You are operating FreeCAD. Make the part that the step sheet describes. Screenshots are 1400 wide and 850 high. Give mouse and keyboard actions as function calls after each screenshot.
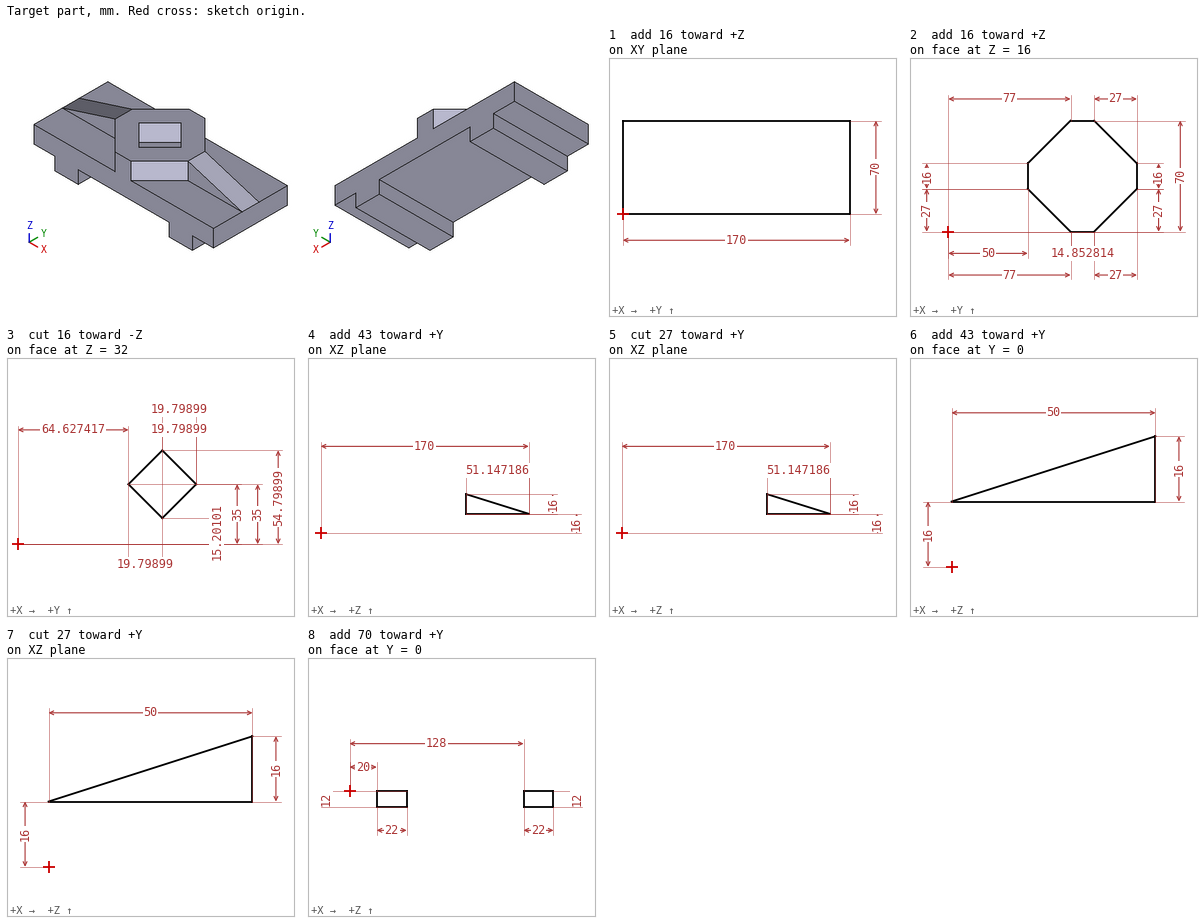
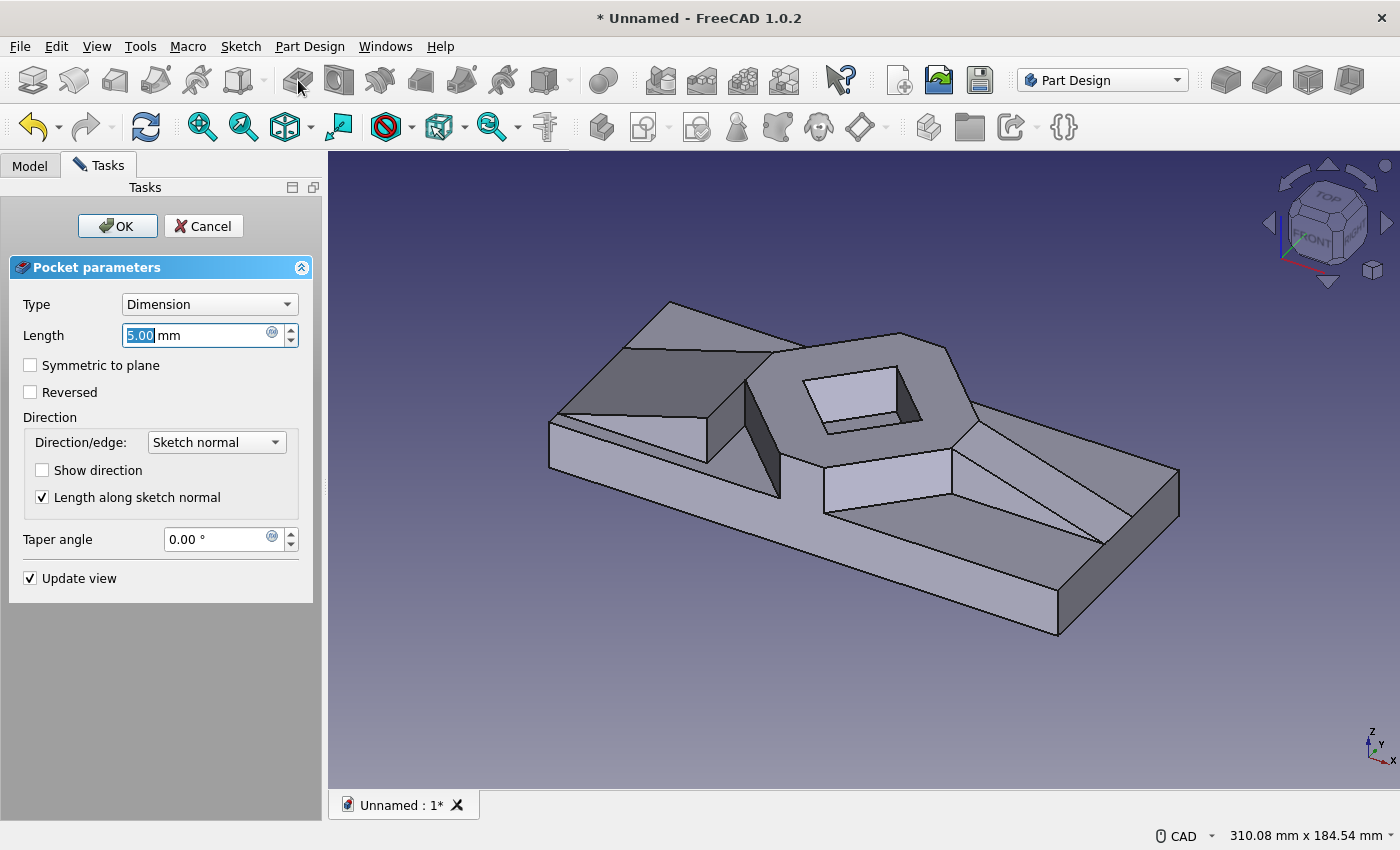
text(27)
key(Tab)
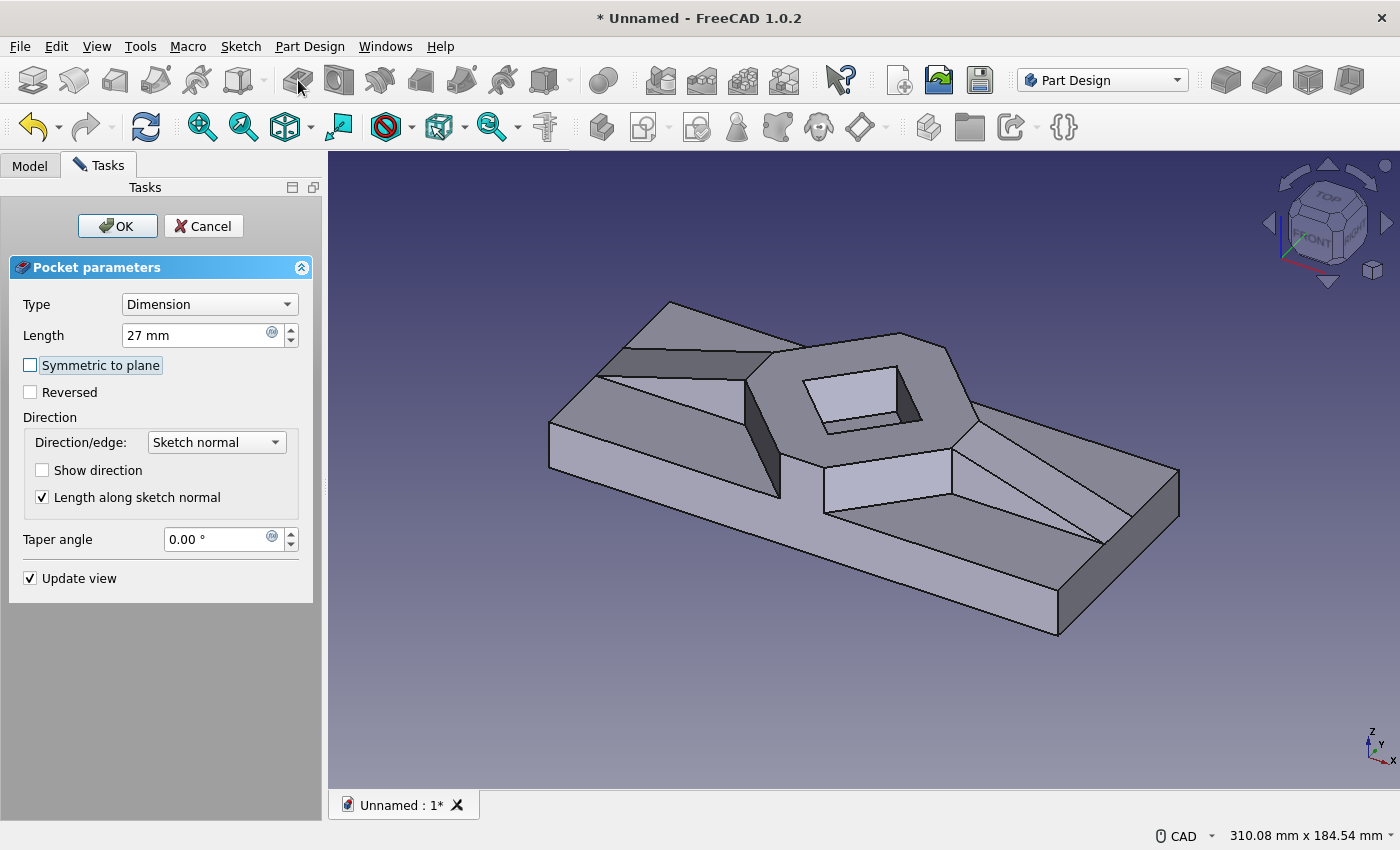
click(118, 226)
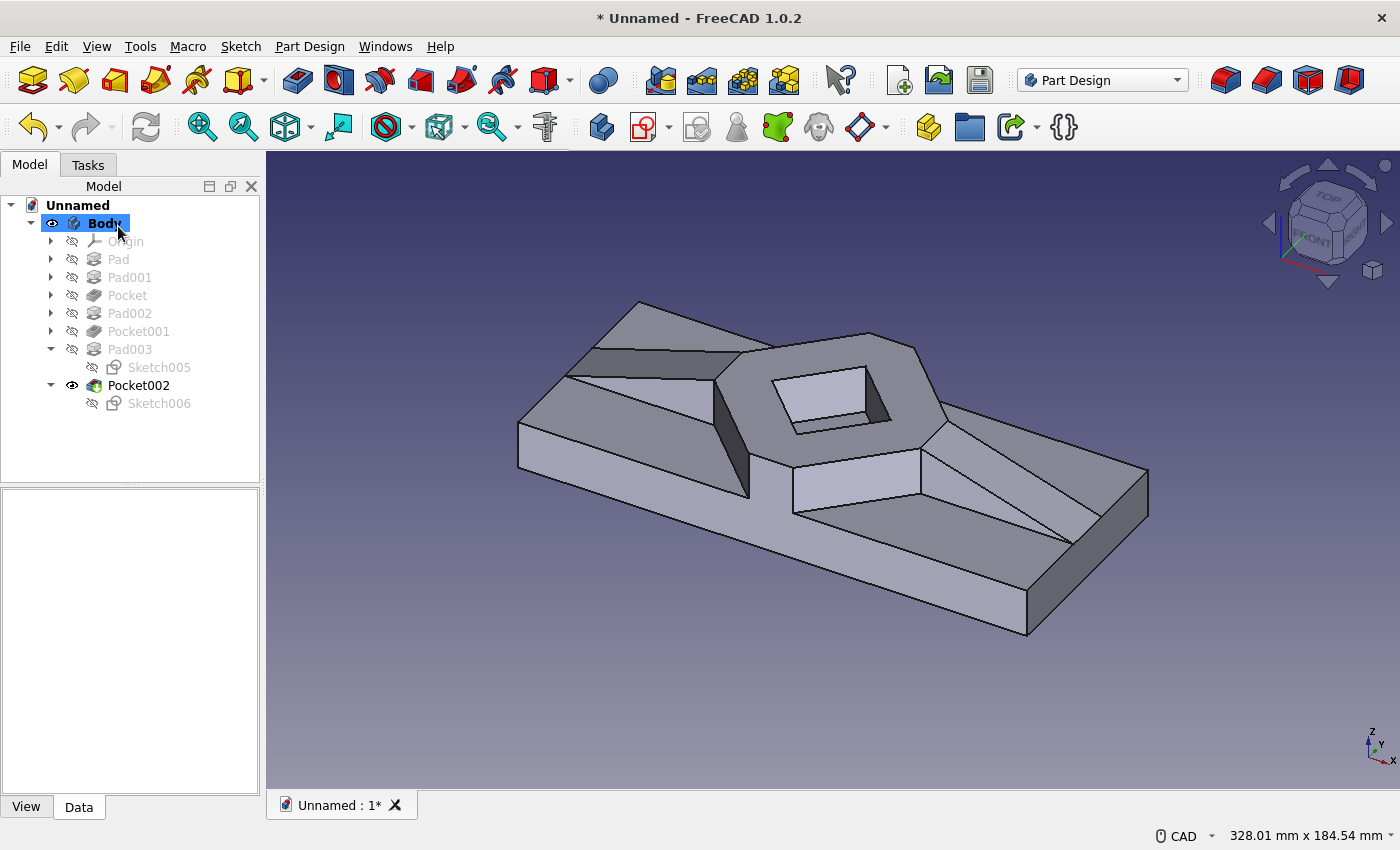
click(772, 518)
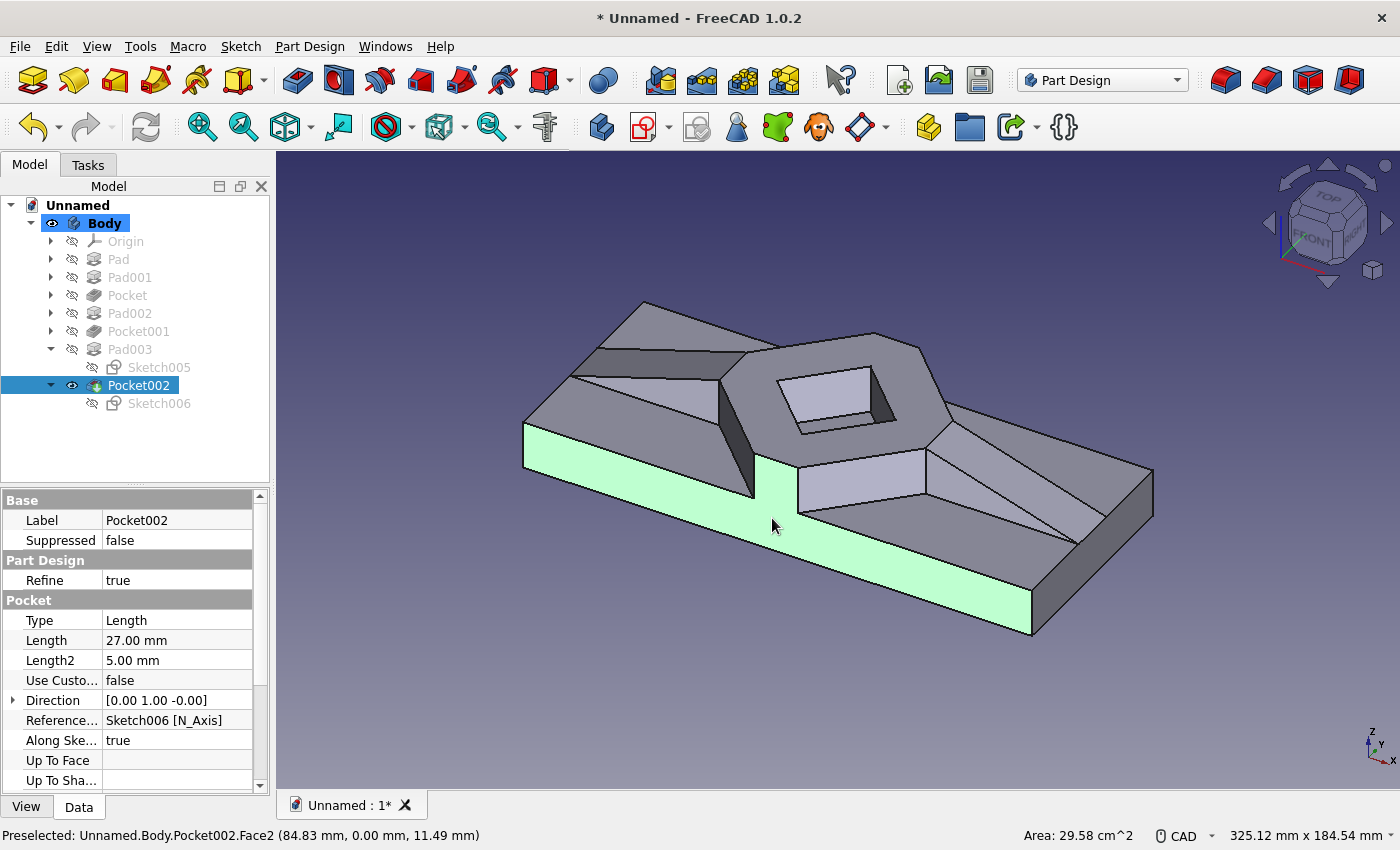
click(642, 128)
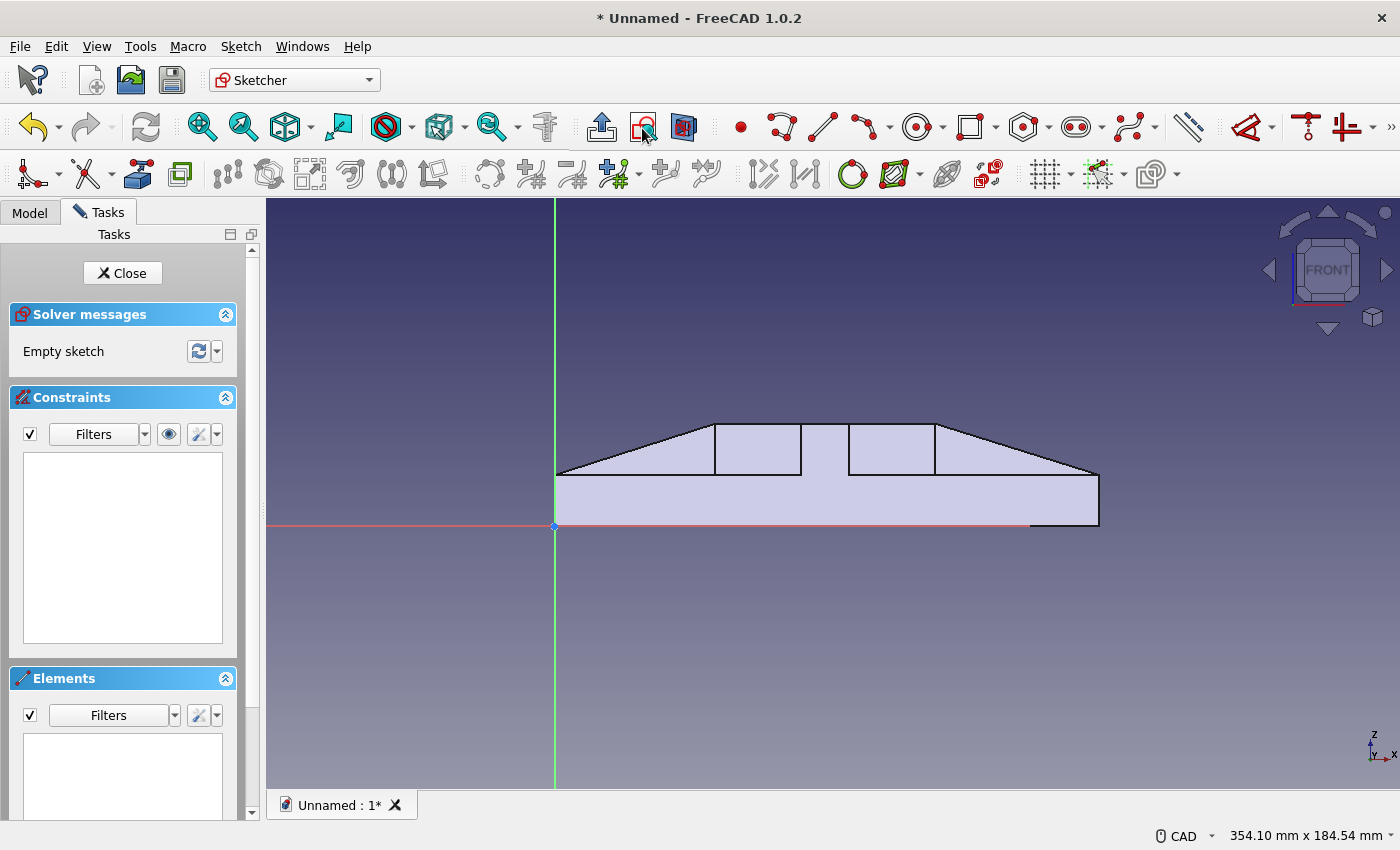
scroll(857, 651, up, 2)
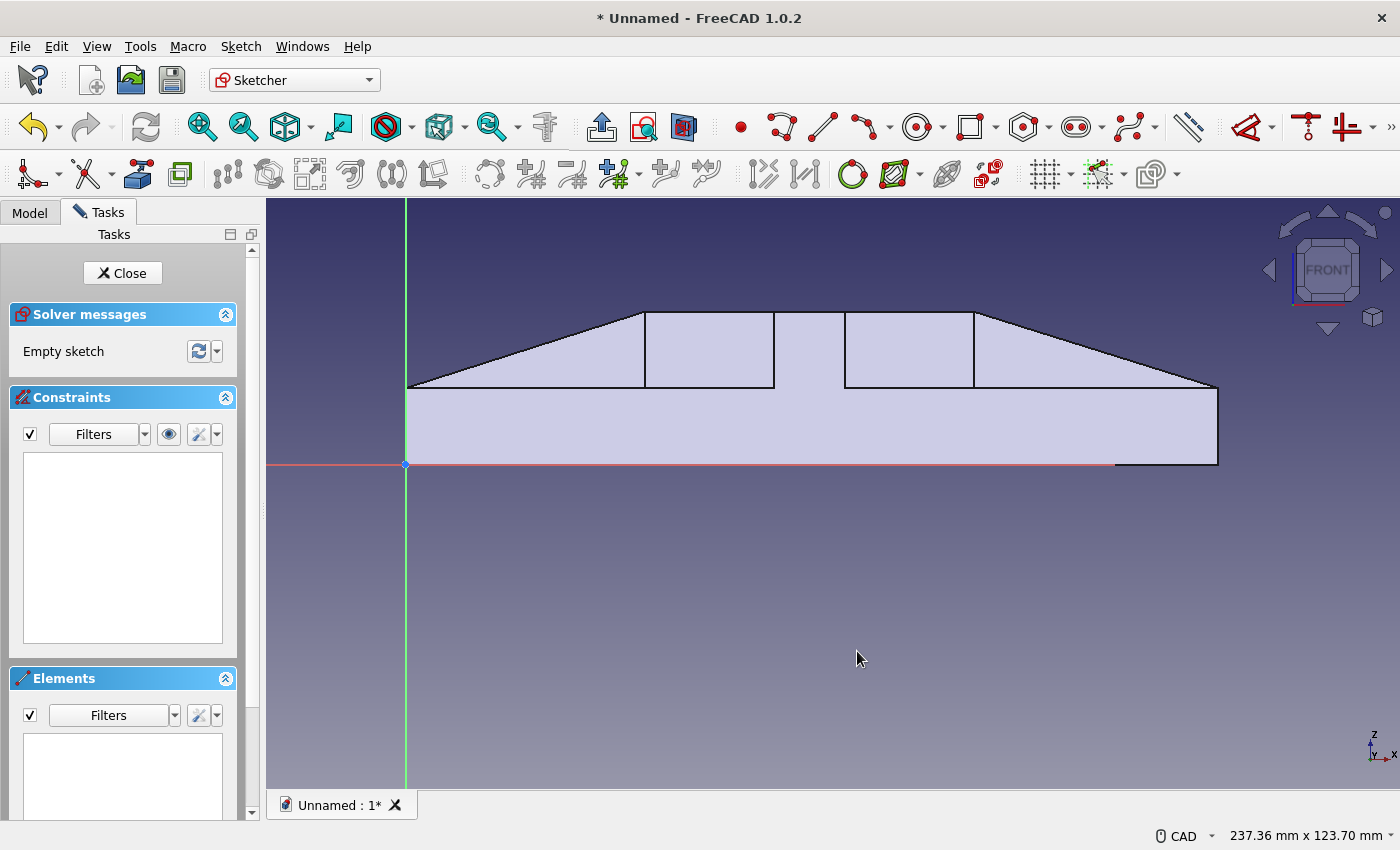
key(g)
key(r)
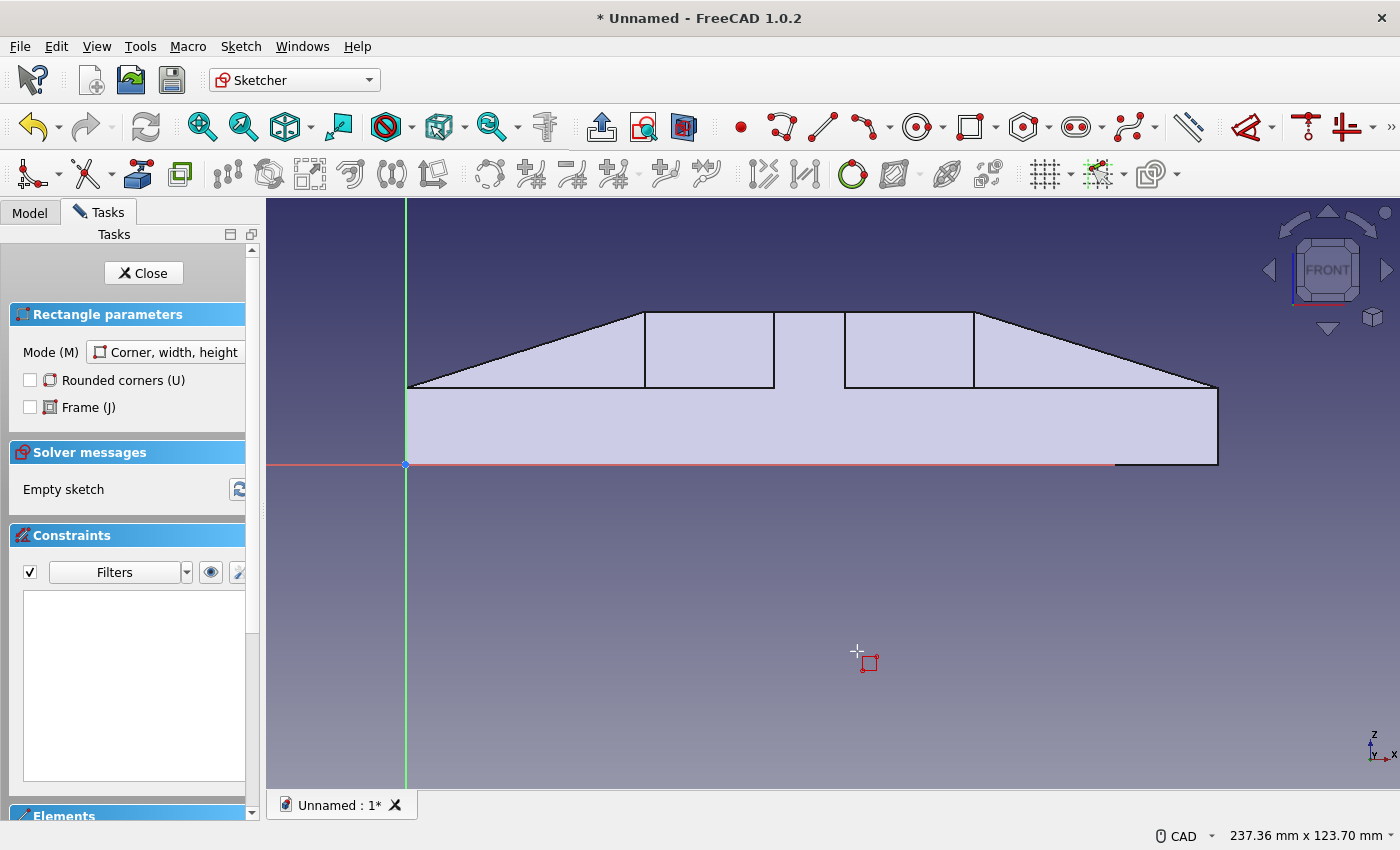
click(501, 465)
move(607, 522)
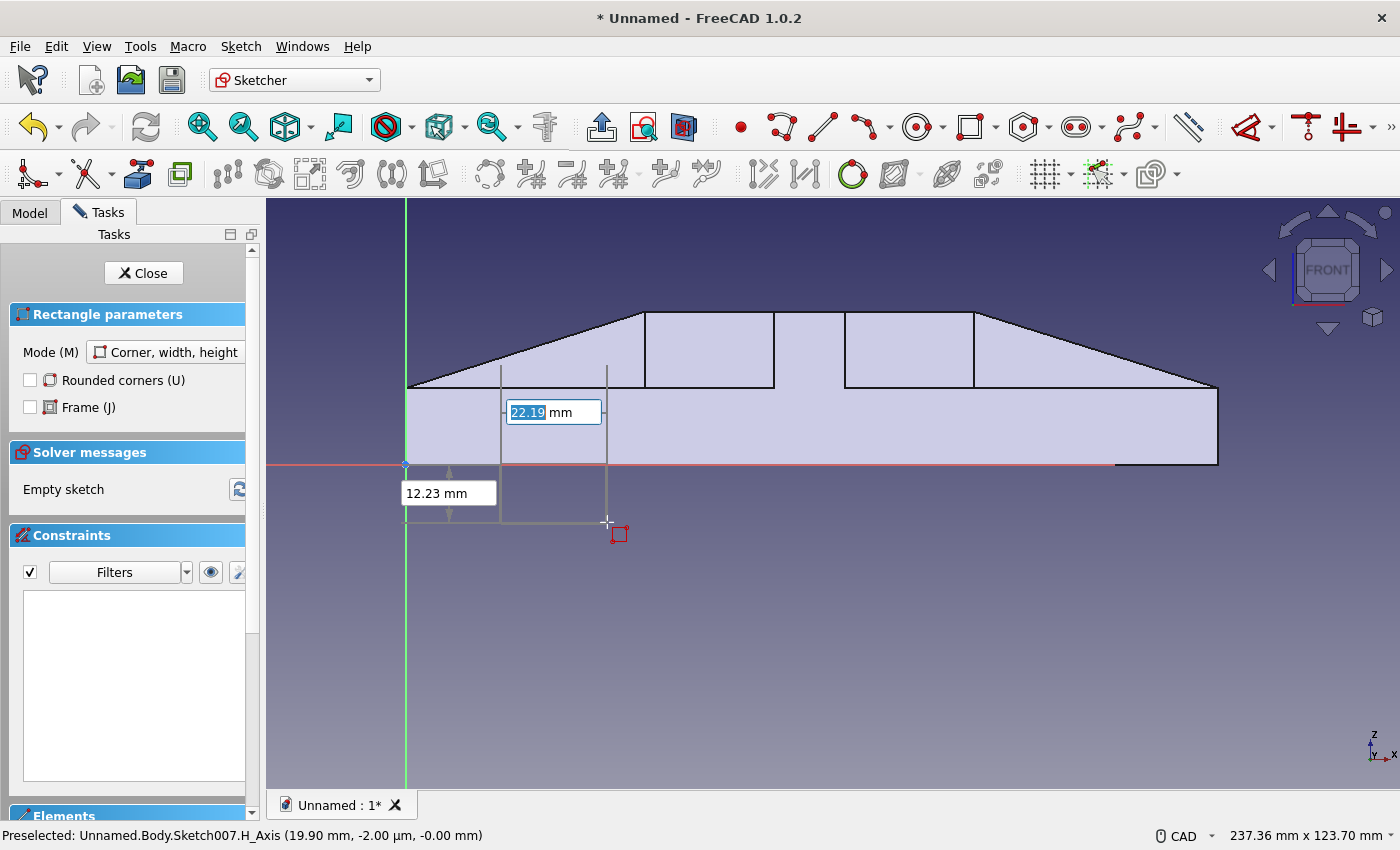
text(22)
key(Tab)
text(12)
key(Return)